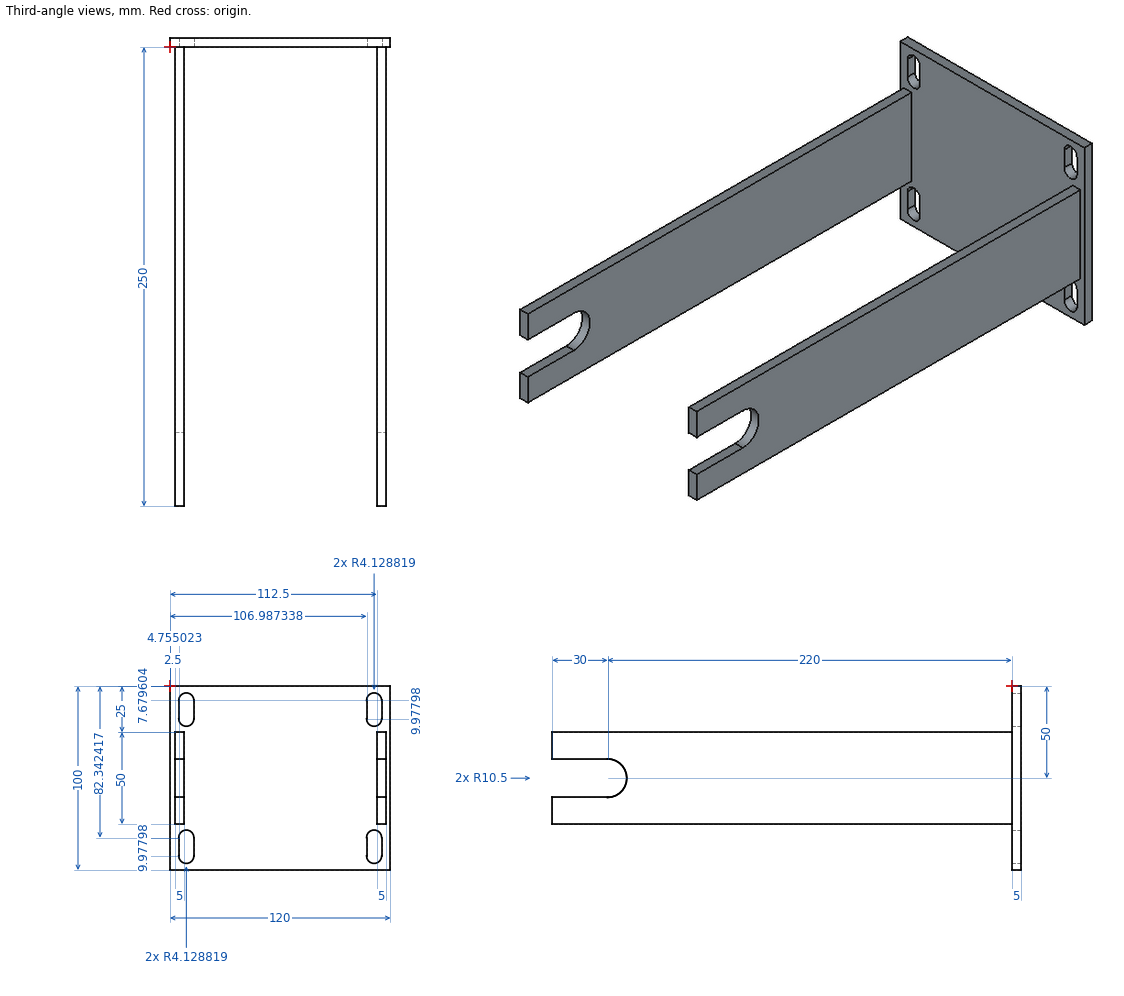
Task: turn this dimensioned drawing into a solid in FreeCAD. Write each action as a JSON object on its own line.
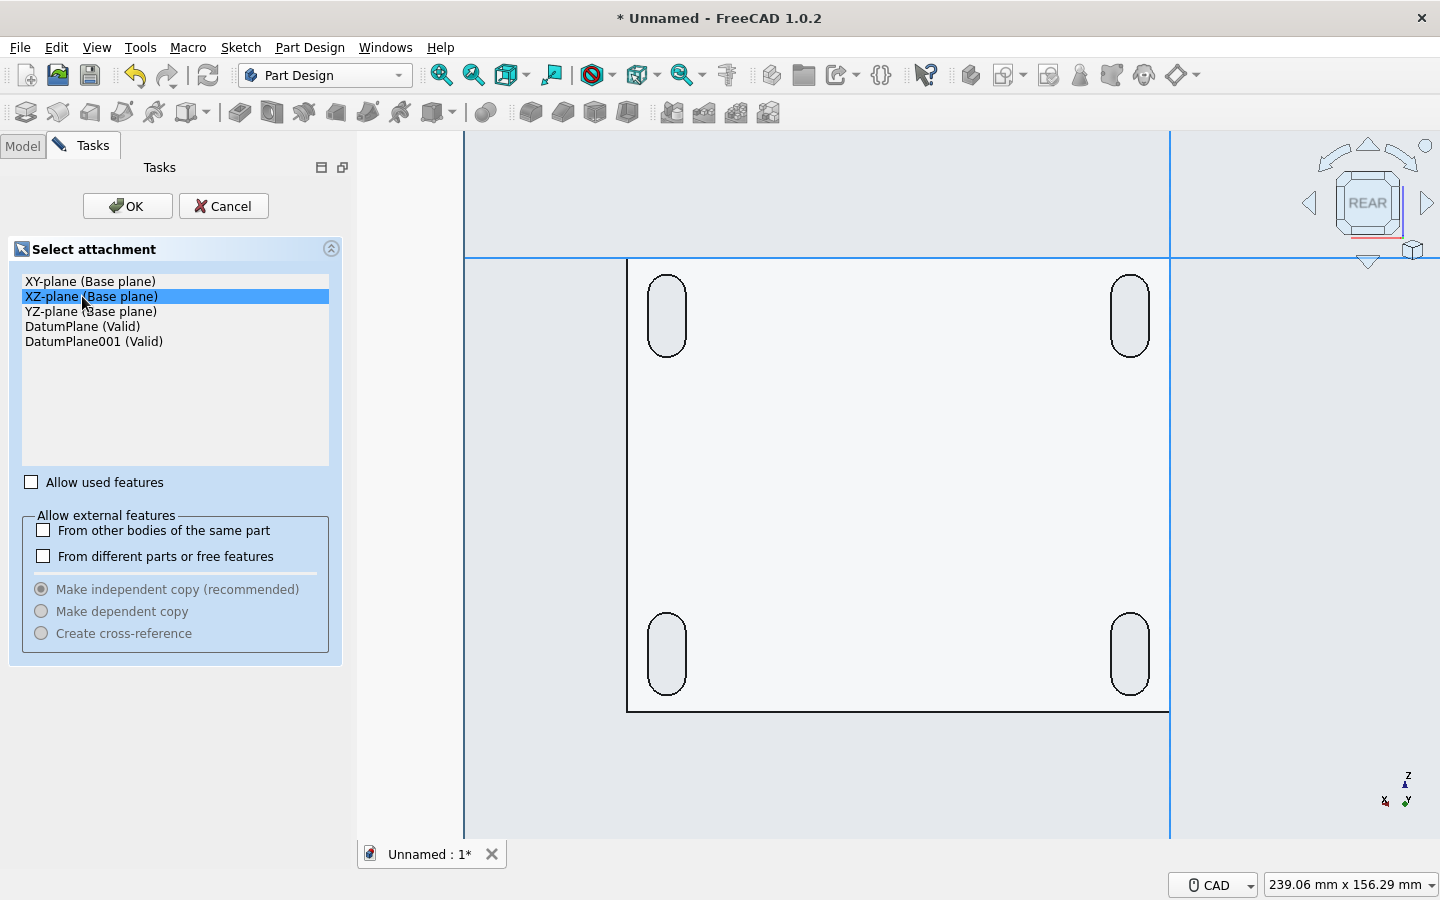
{"action": "left_click", "coordinate": [128, 206]}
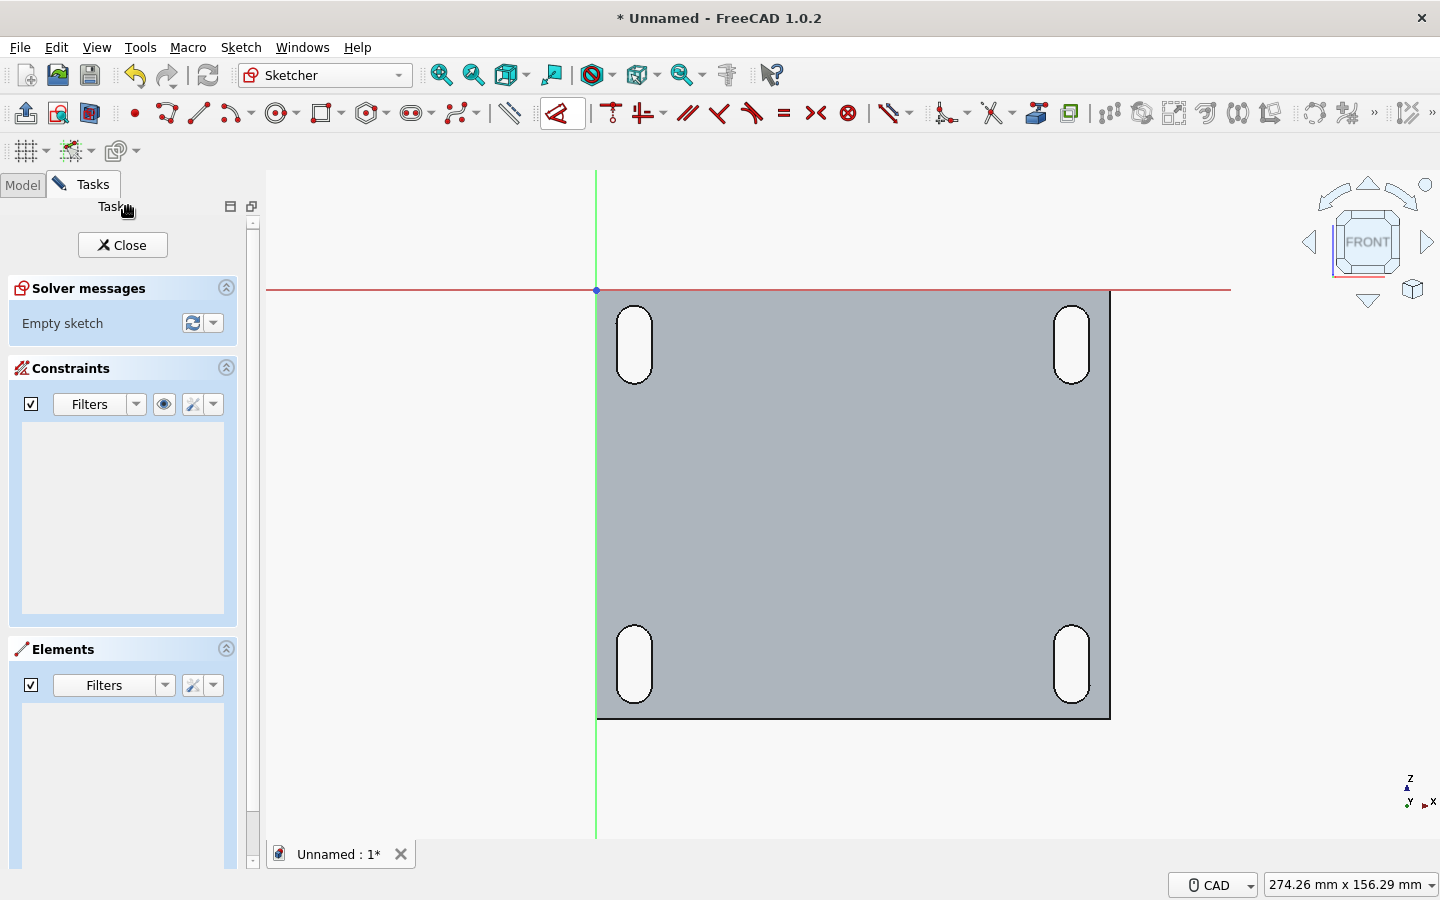
{"action": "key", "text": "g r"}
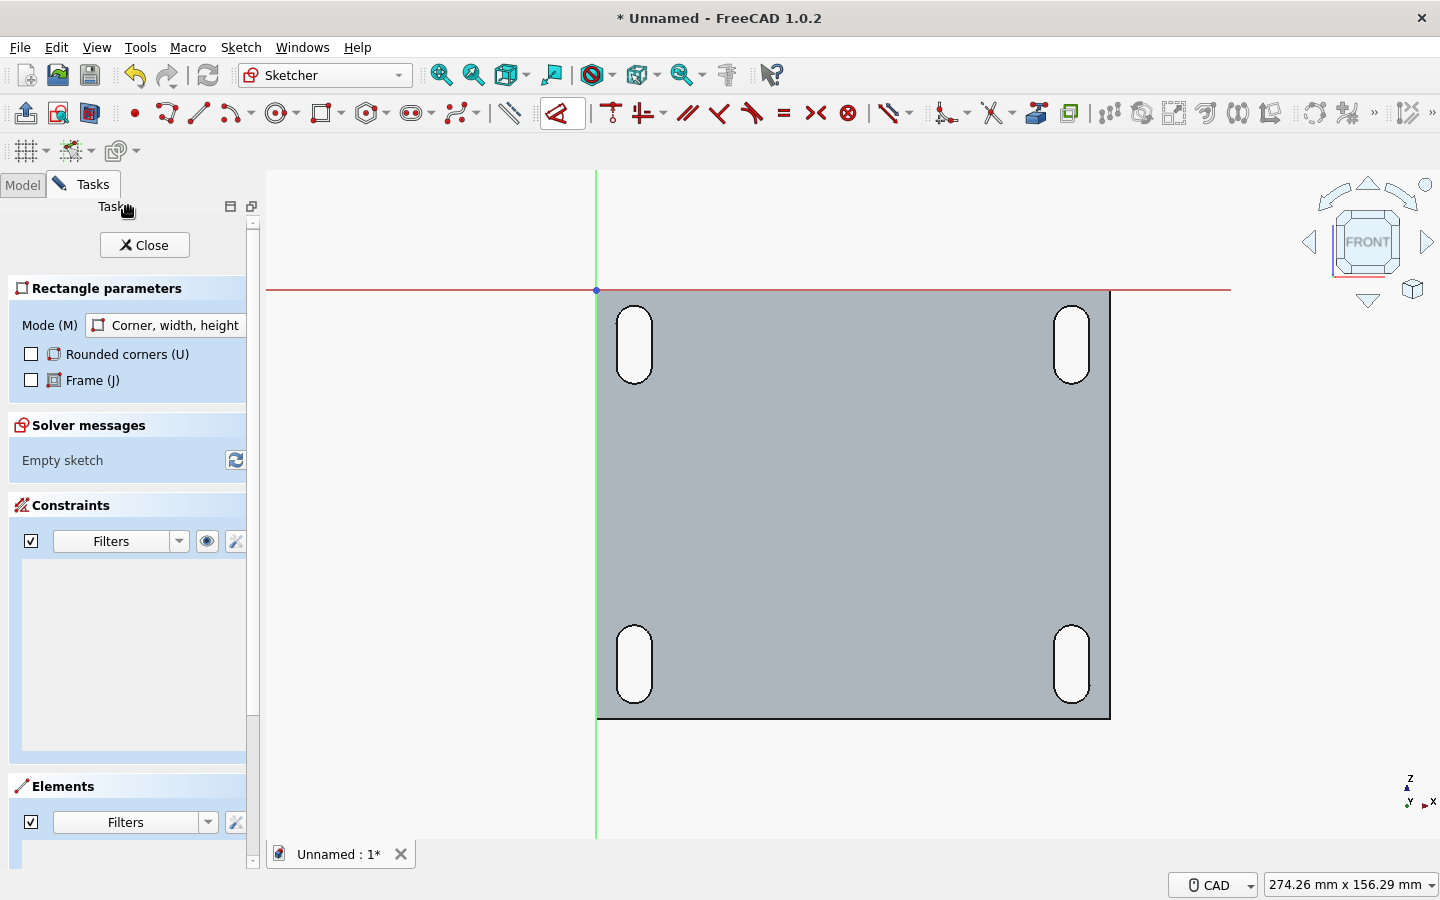
{"action": "scroll", "coordinate": [607, 397], "scroll_direction": "up", "scroll_amount": 2}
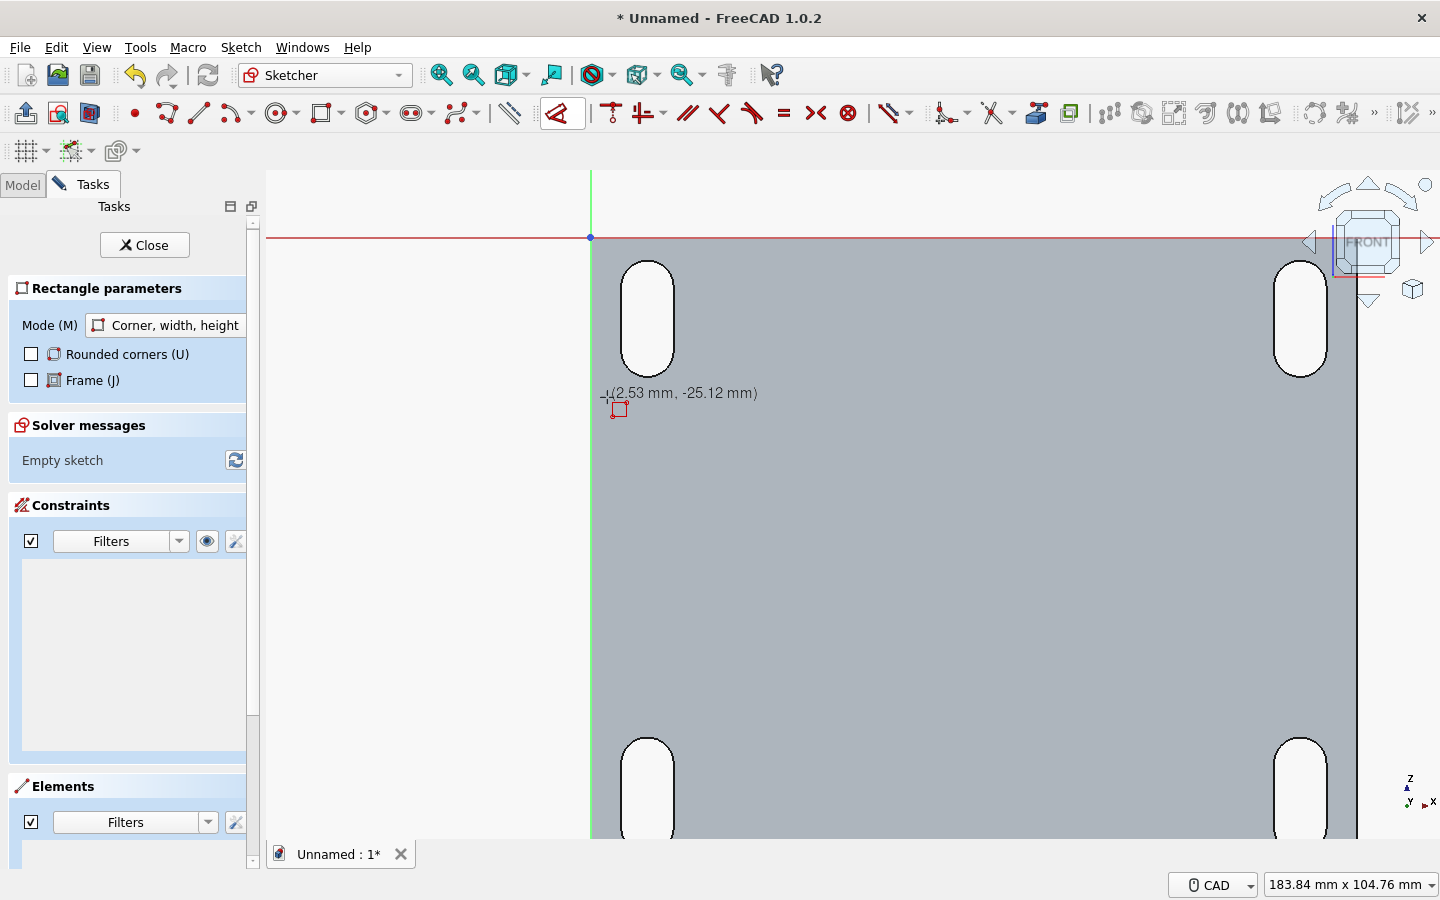
{"action": "left_click", "coordinate": [607, 398]}
{"action": "left_click", "coordinate": [639, 717]}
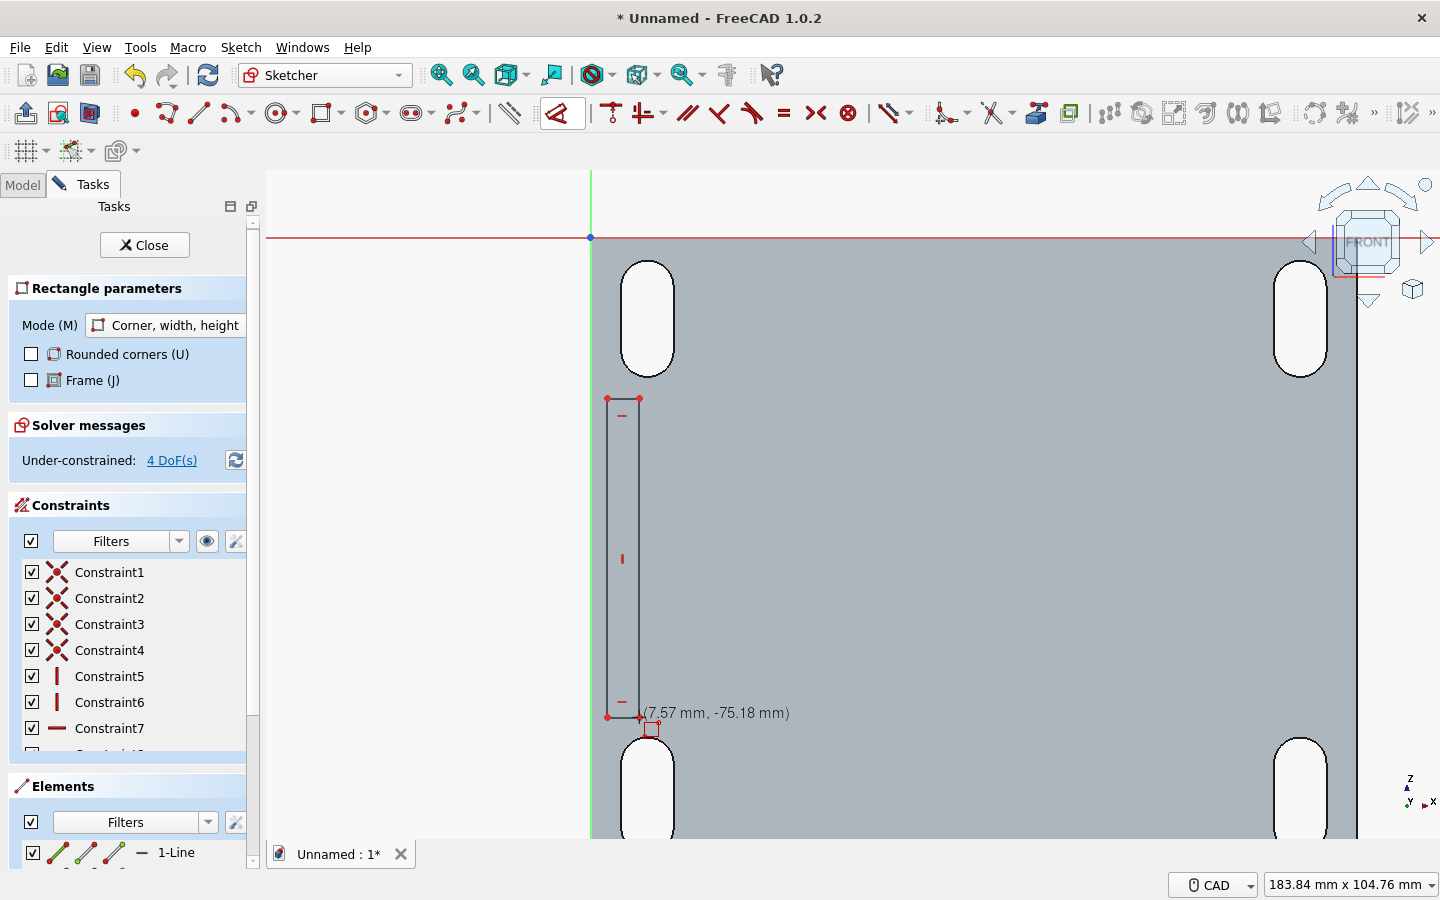
{"action": "scroll", "coordinate": [294, 627], "scroll_direction": "down", "scroll_amount": 1}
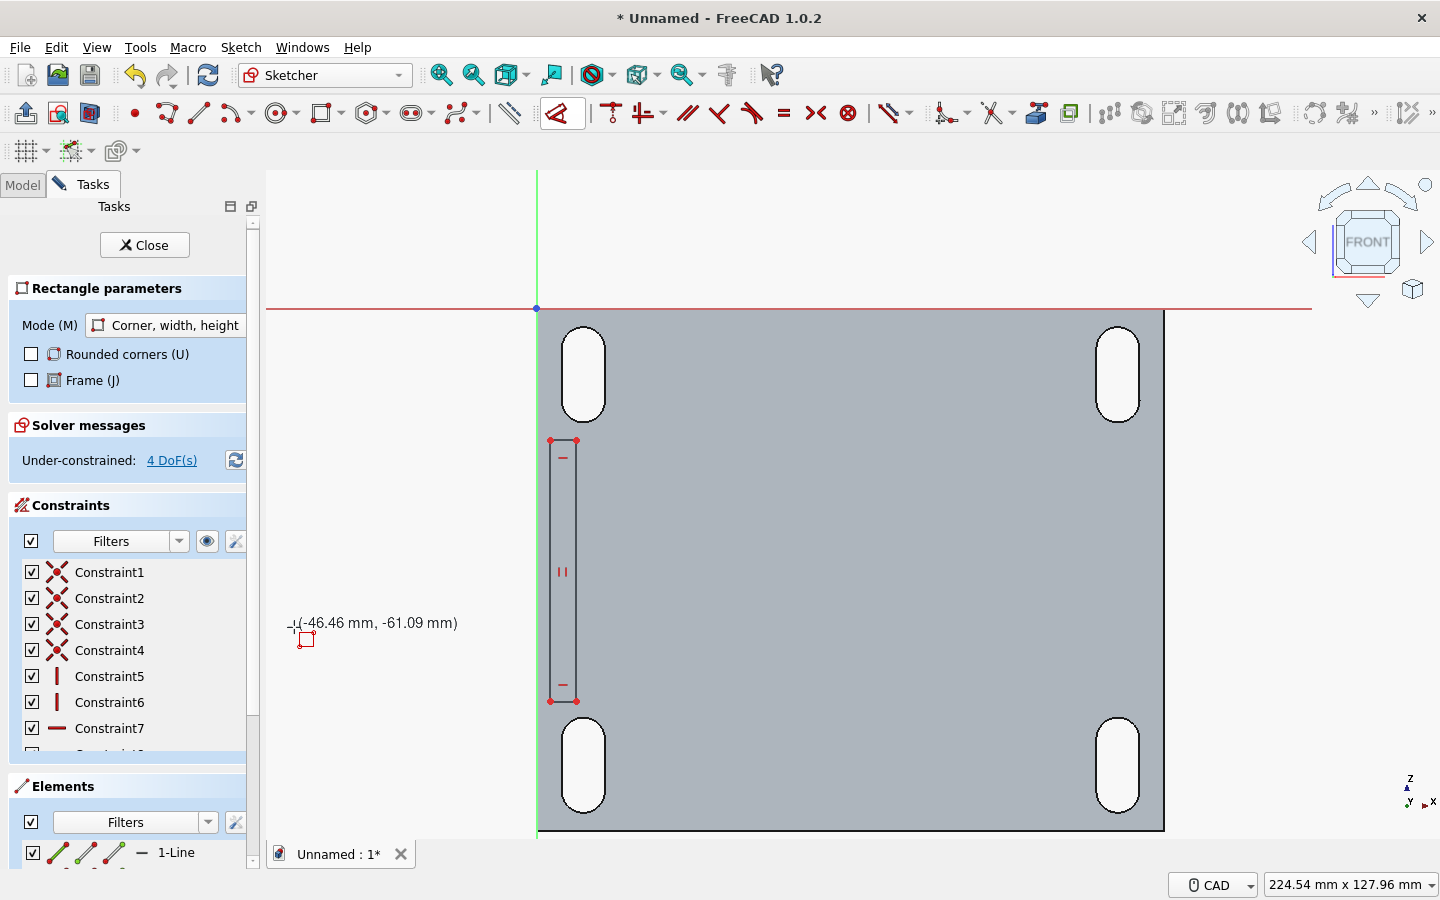
{"action": "left_click", "coordinate": [1125, 439]}
{"action": "left_click", "coordinate": [1151, 701]}
{"action": "key", "text": "Escape"}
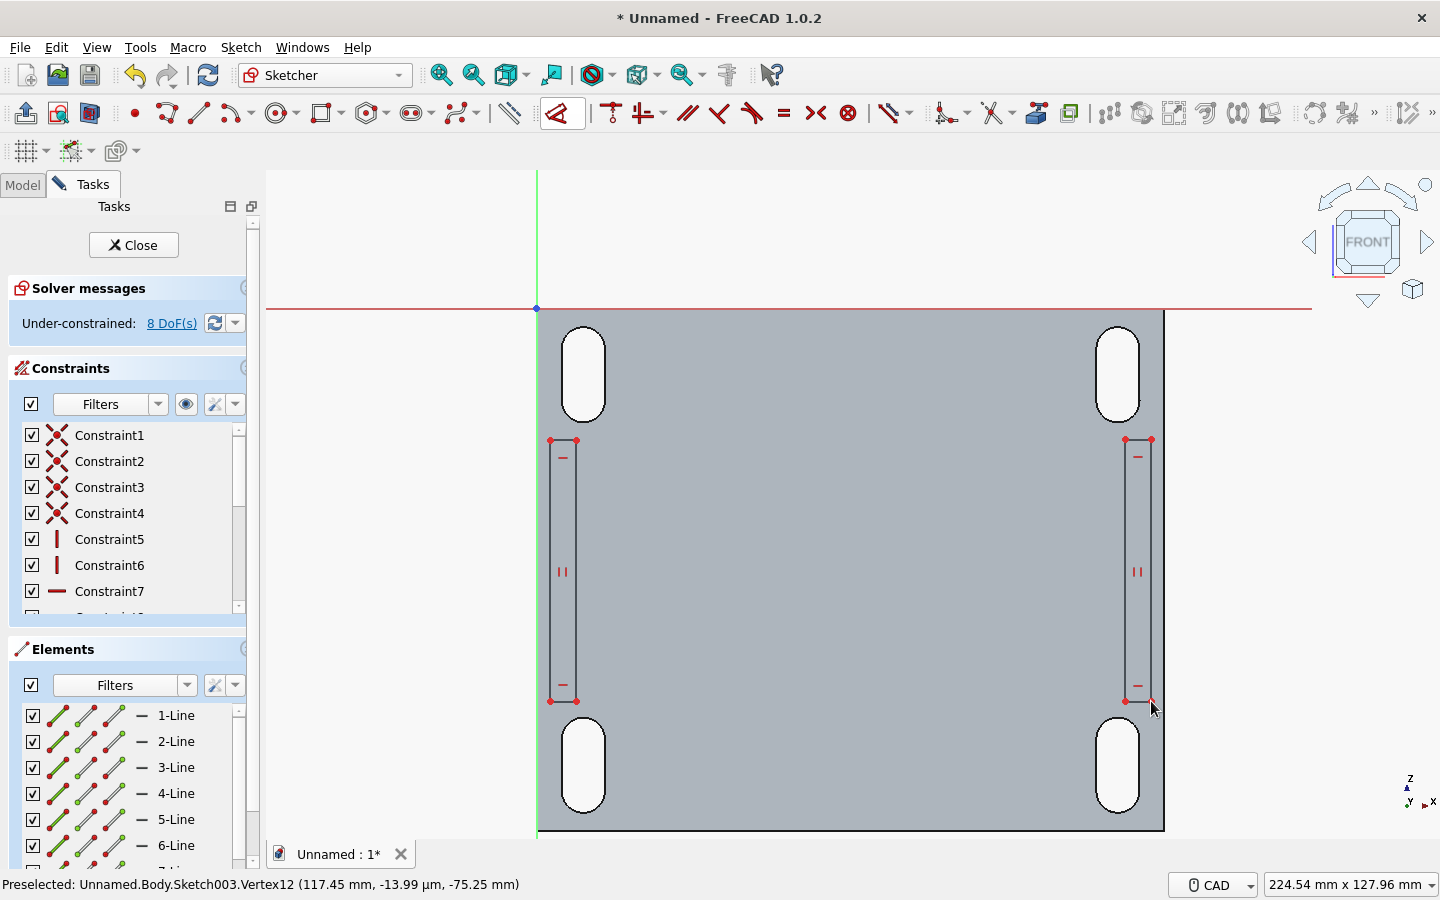
{"action": "scroll", "coordinate": [561, 702], "scroll_direction": "up", "scroll_amount": 3}